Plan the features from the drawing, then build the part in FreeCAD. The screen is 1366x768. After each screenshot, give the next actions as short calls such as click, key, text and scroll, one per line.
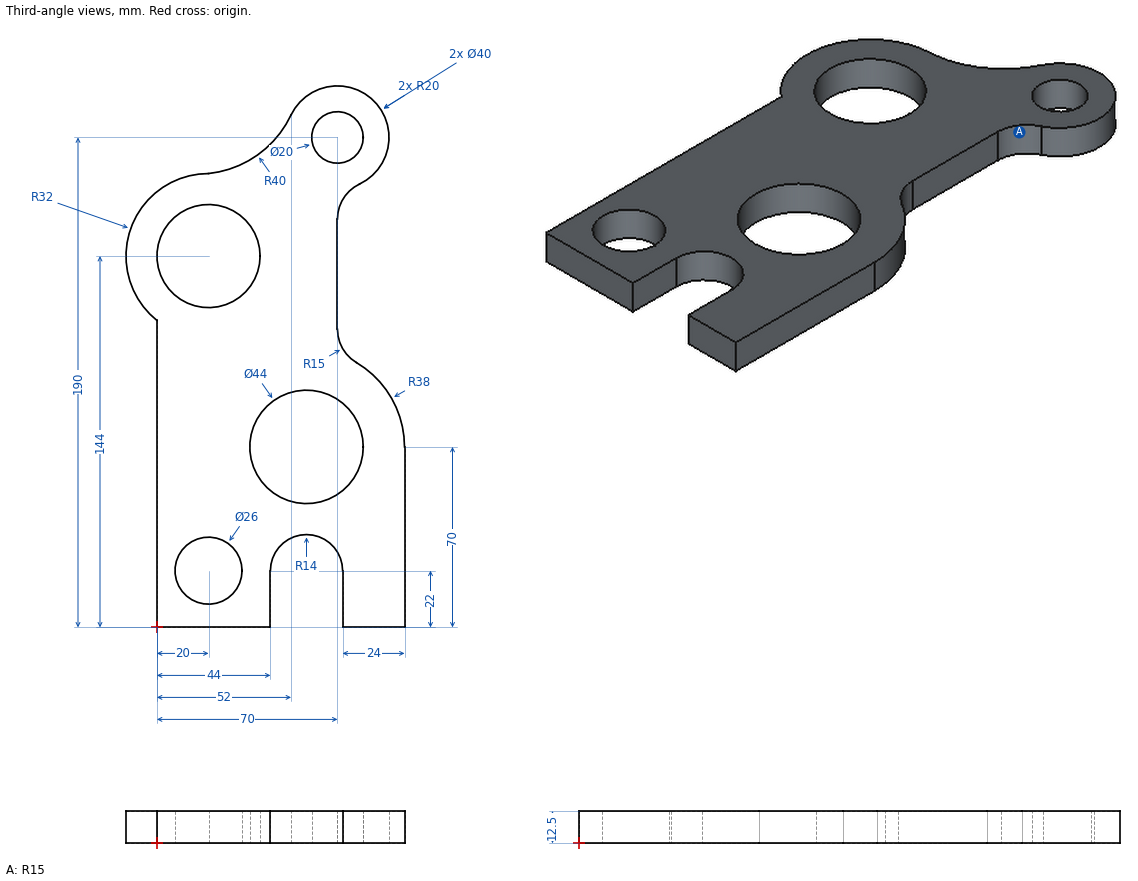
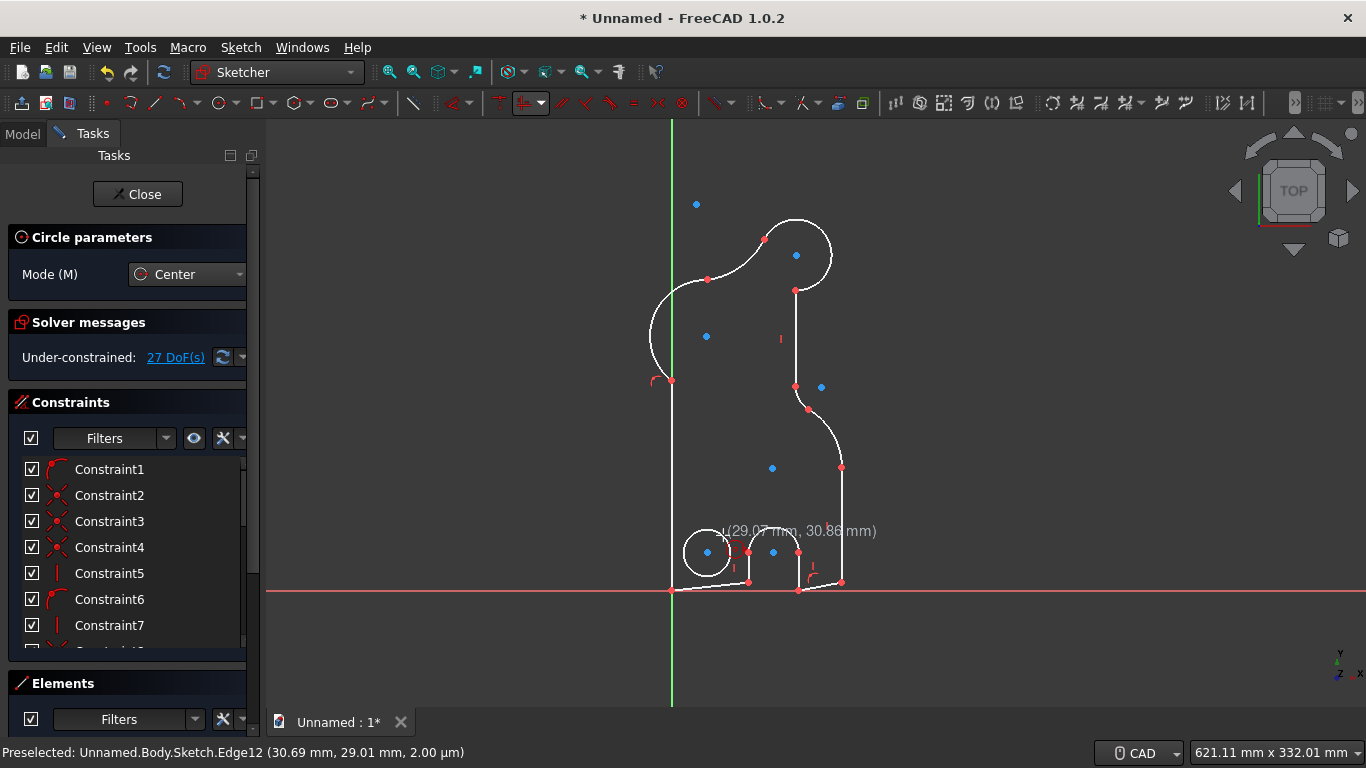
click(774, 467)
click(802, 439)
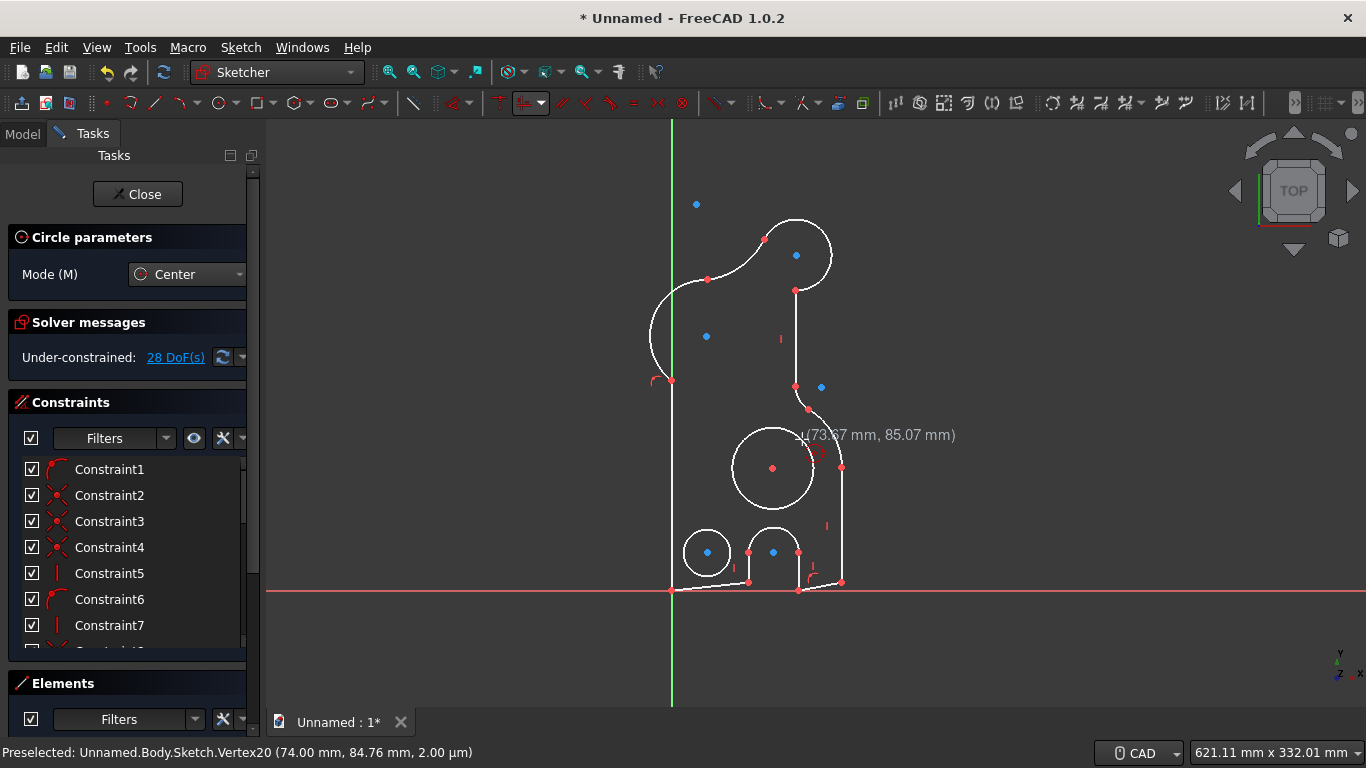
click(707, 336)
click(732, 311)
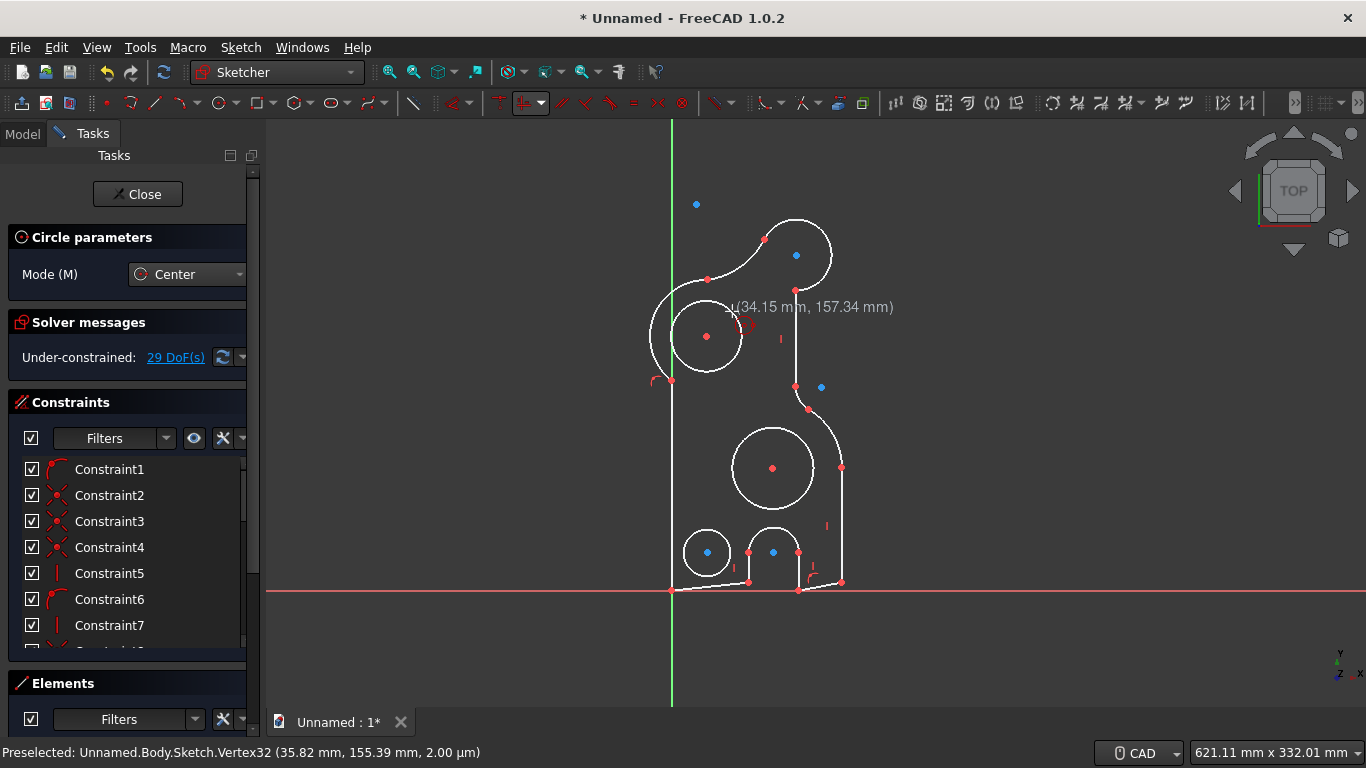
scroll(795, 254, up, 2)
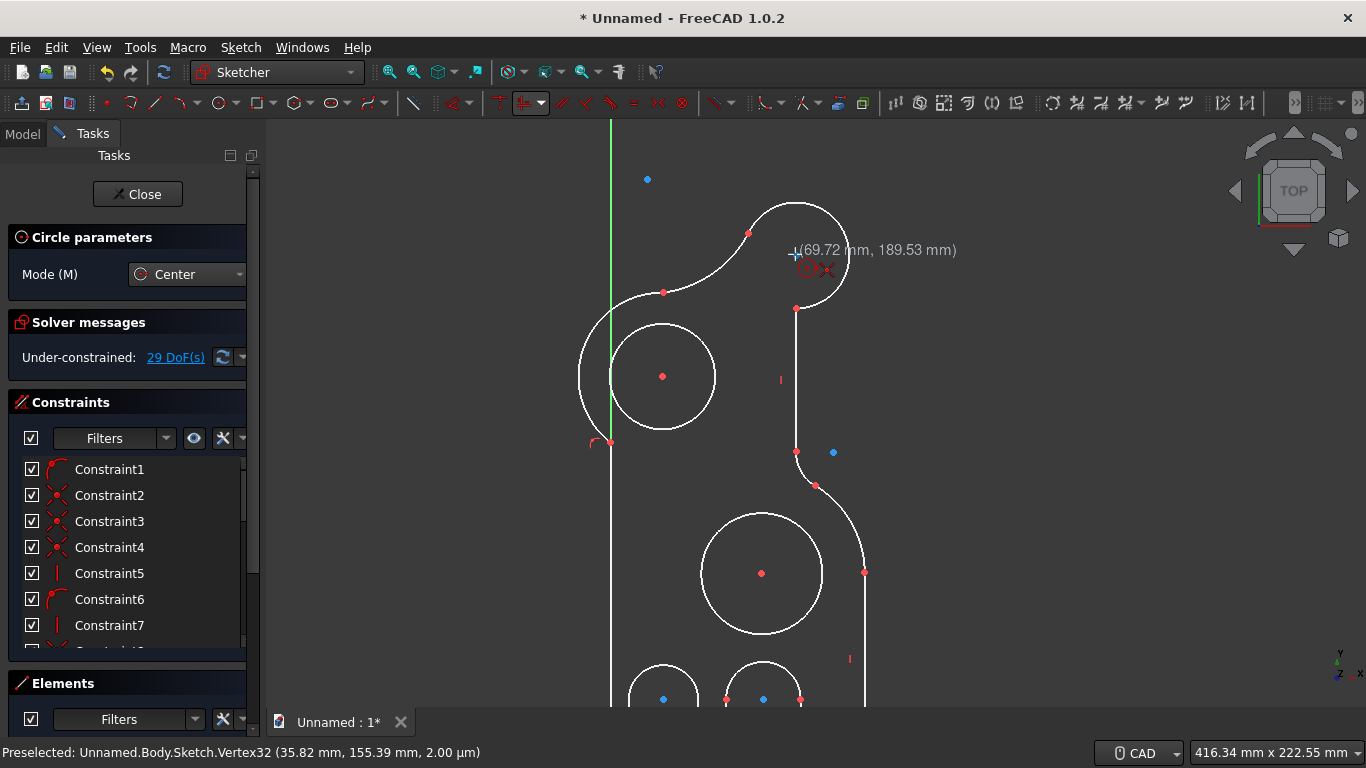
click(796, 254)
click(814, 235)
key(Escape)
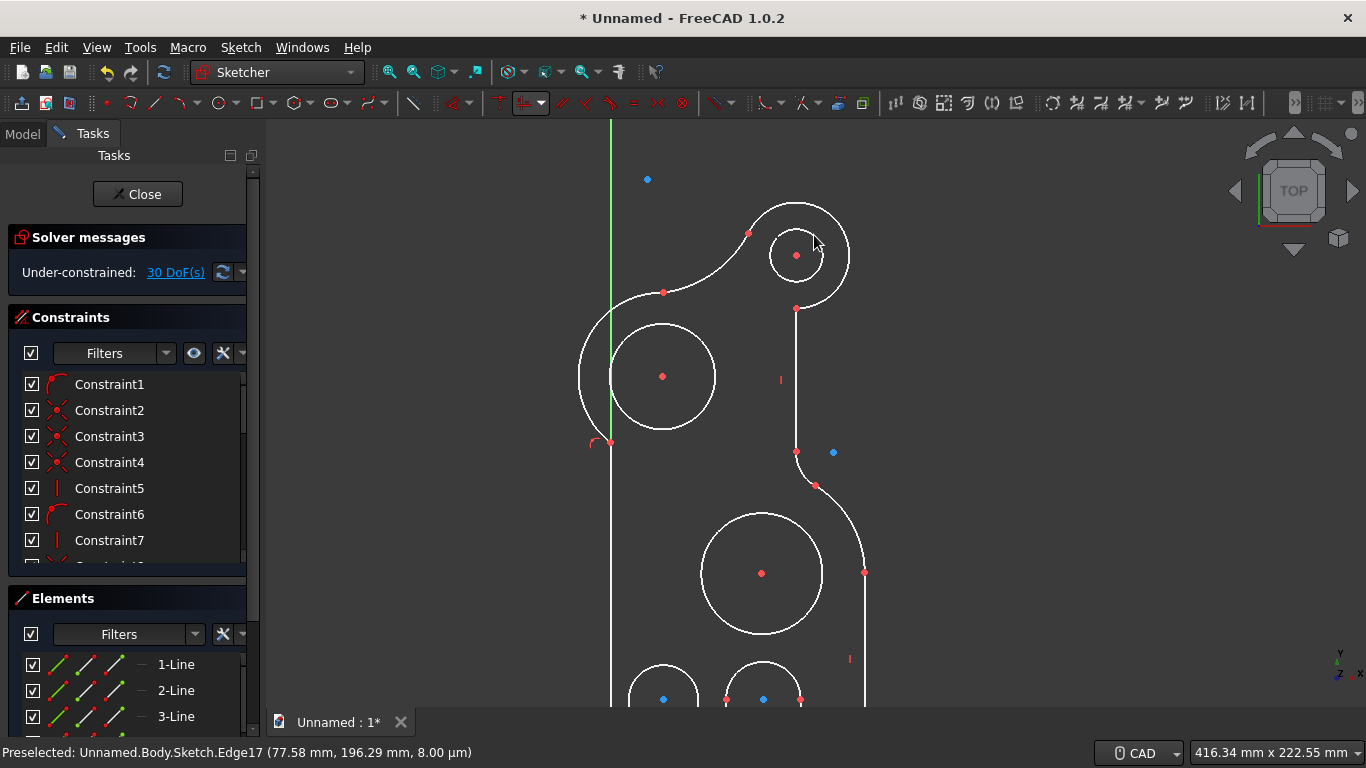
scroll(795, 254, down, 2)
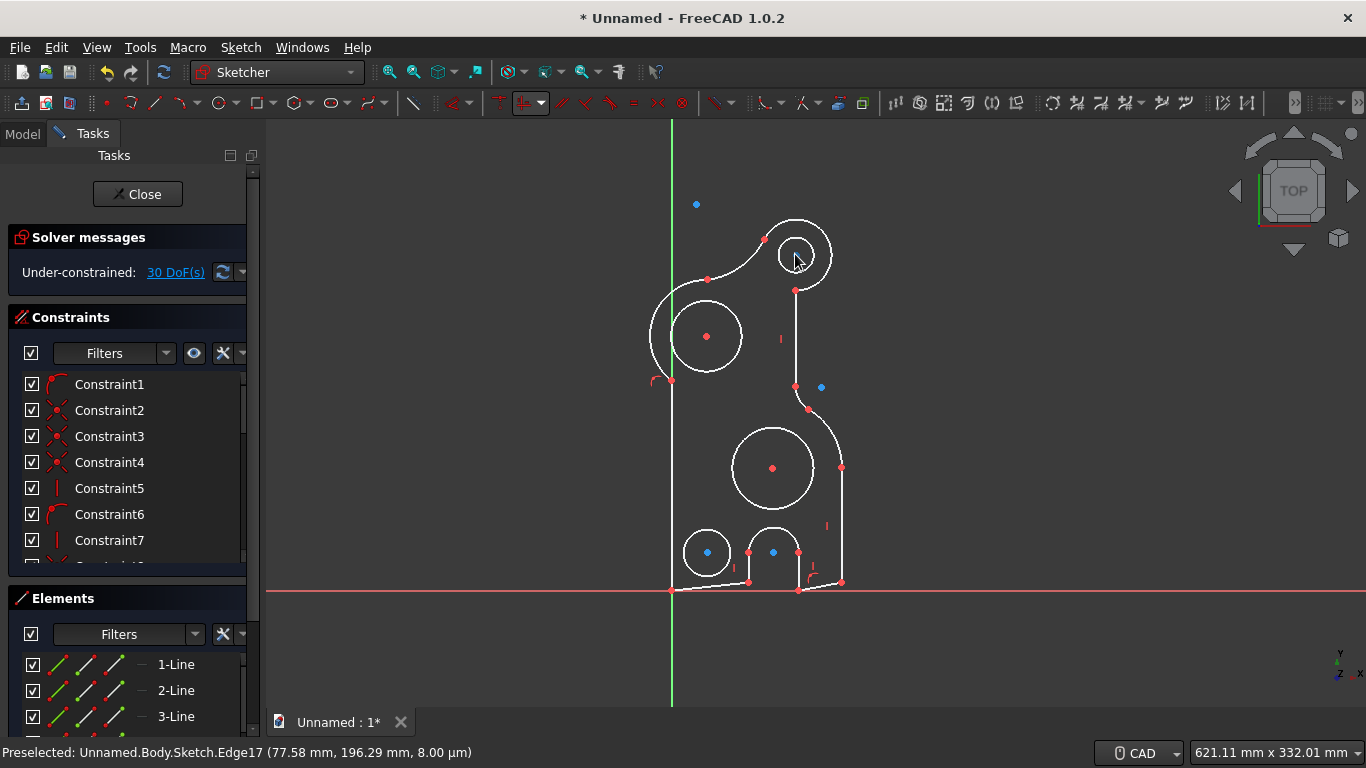
scroll(749, 574, up, 3)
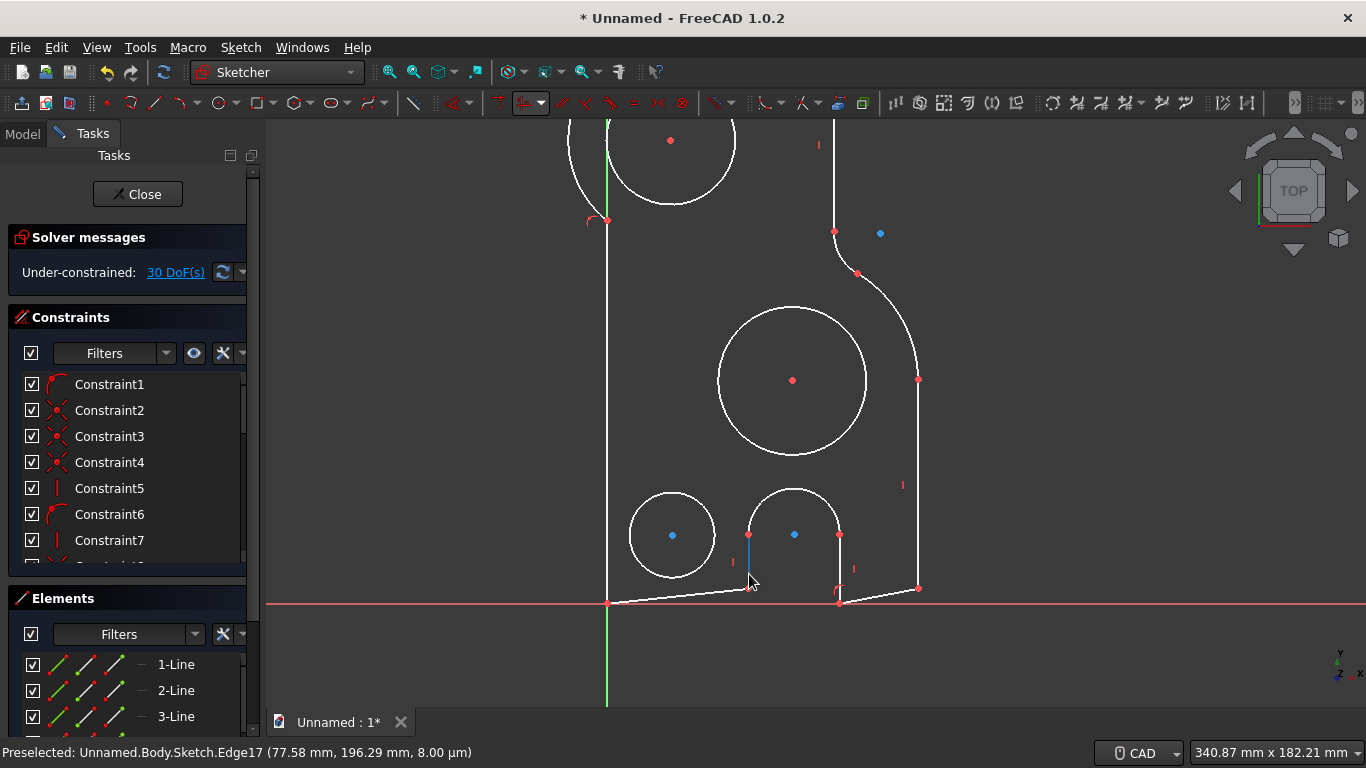
click(749, 572)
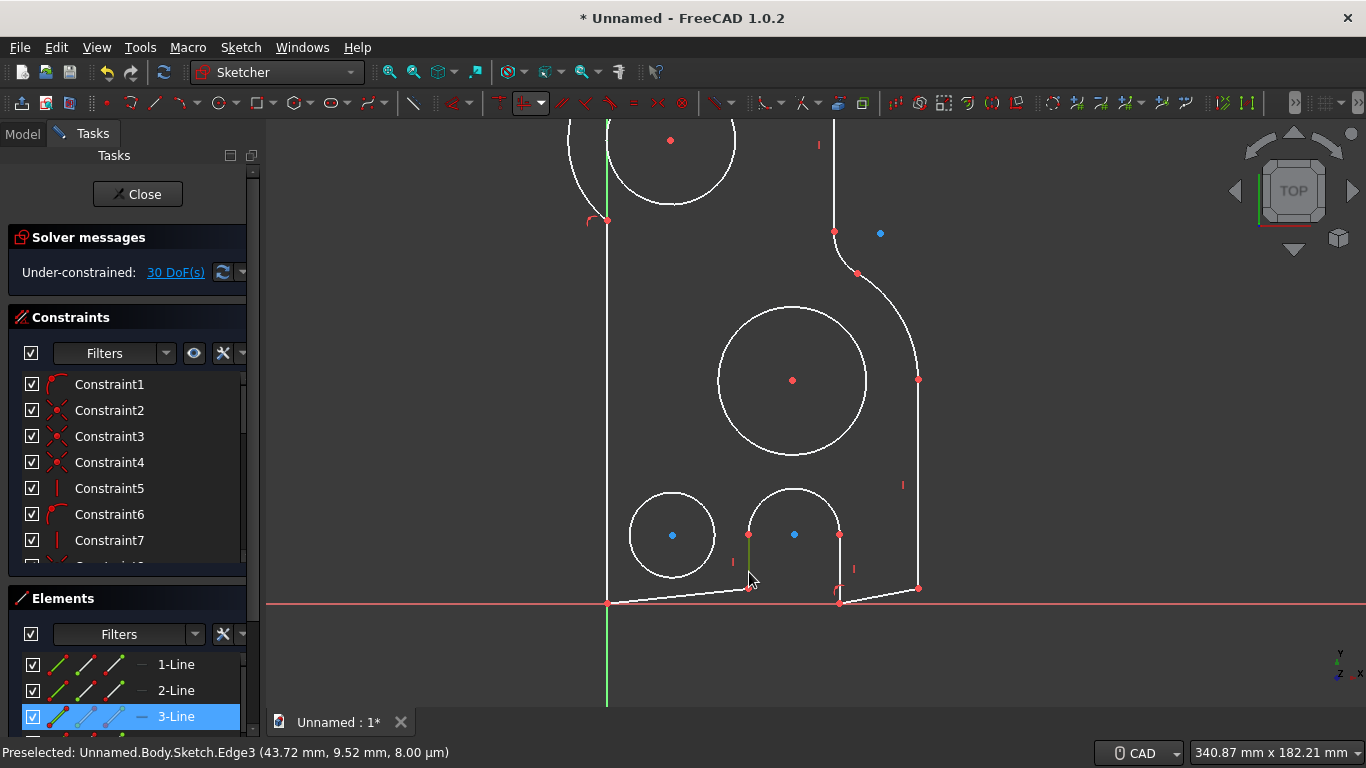
click(821, 497)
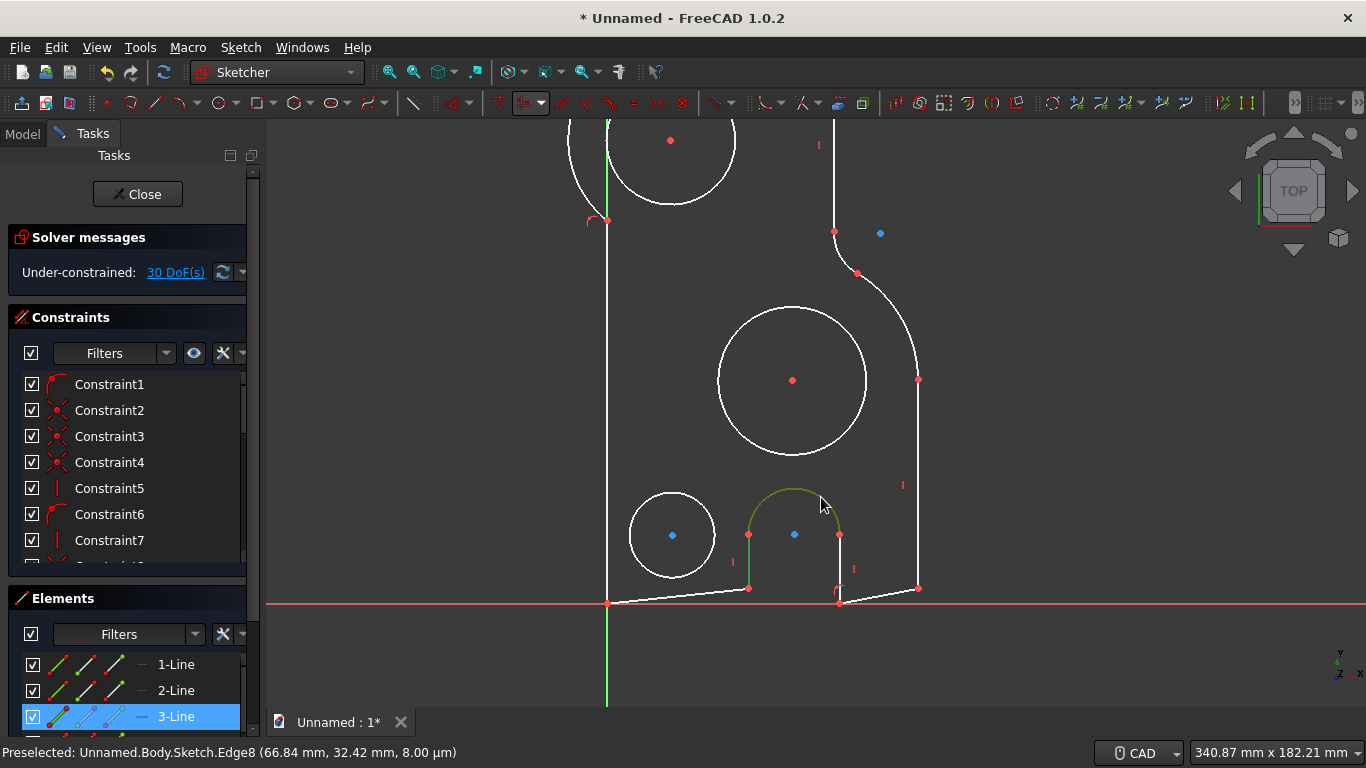
click(610, 104)